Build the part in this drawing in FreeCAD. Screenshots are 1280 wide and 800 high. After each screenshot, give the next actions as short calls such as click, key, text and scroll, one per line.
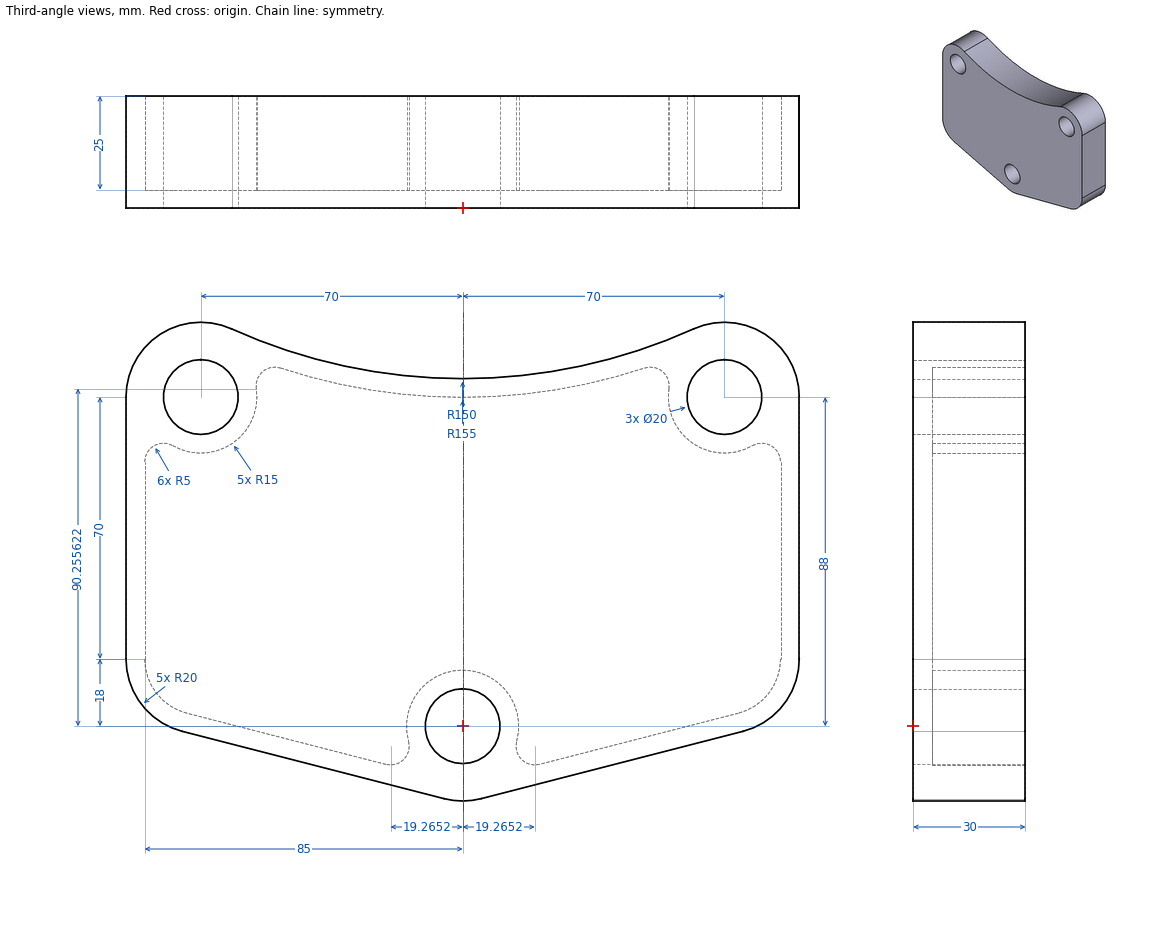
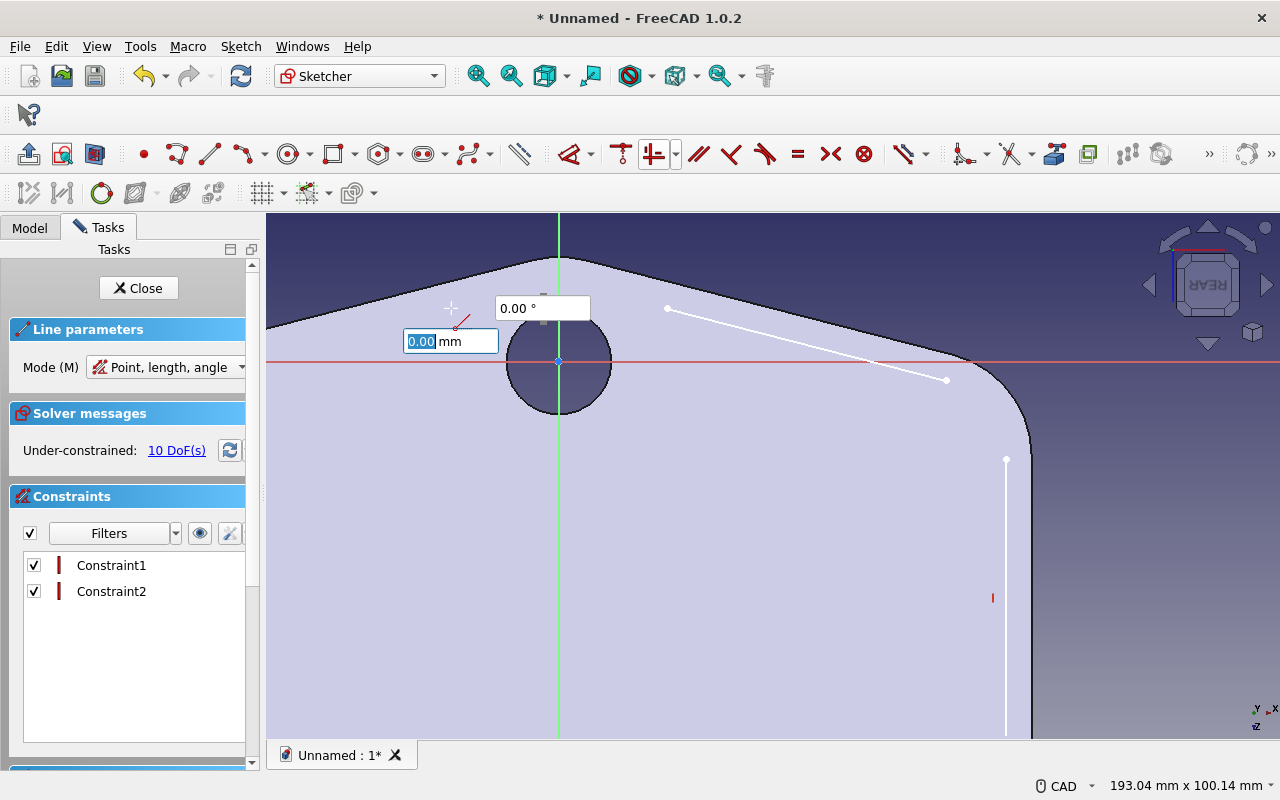
scroll(882, 341, down, 3)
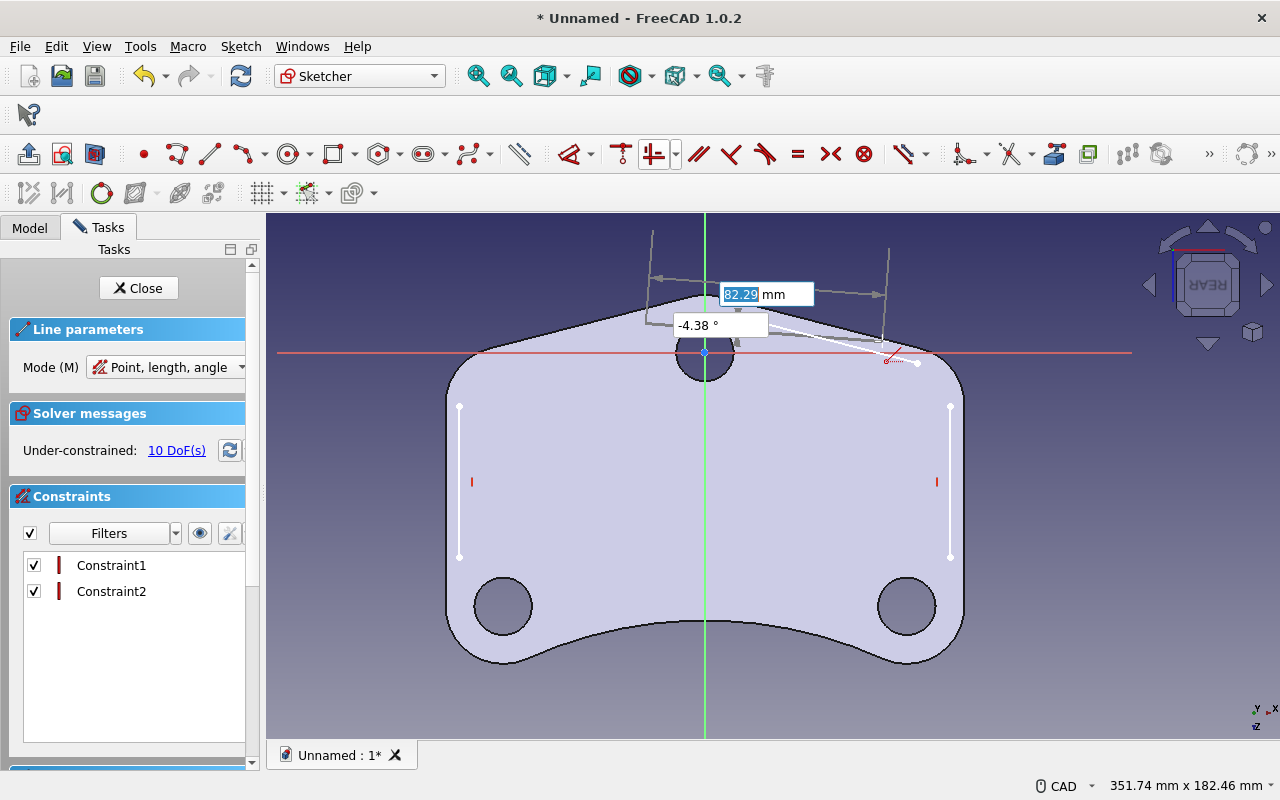
scroll(492, 363, up, 3)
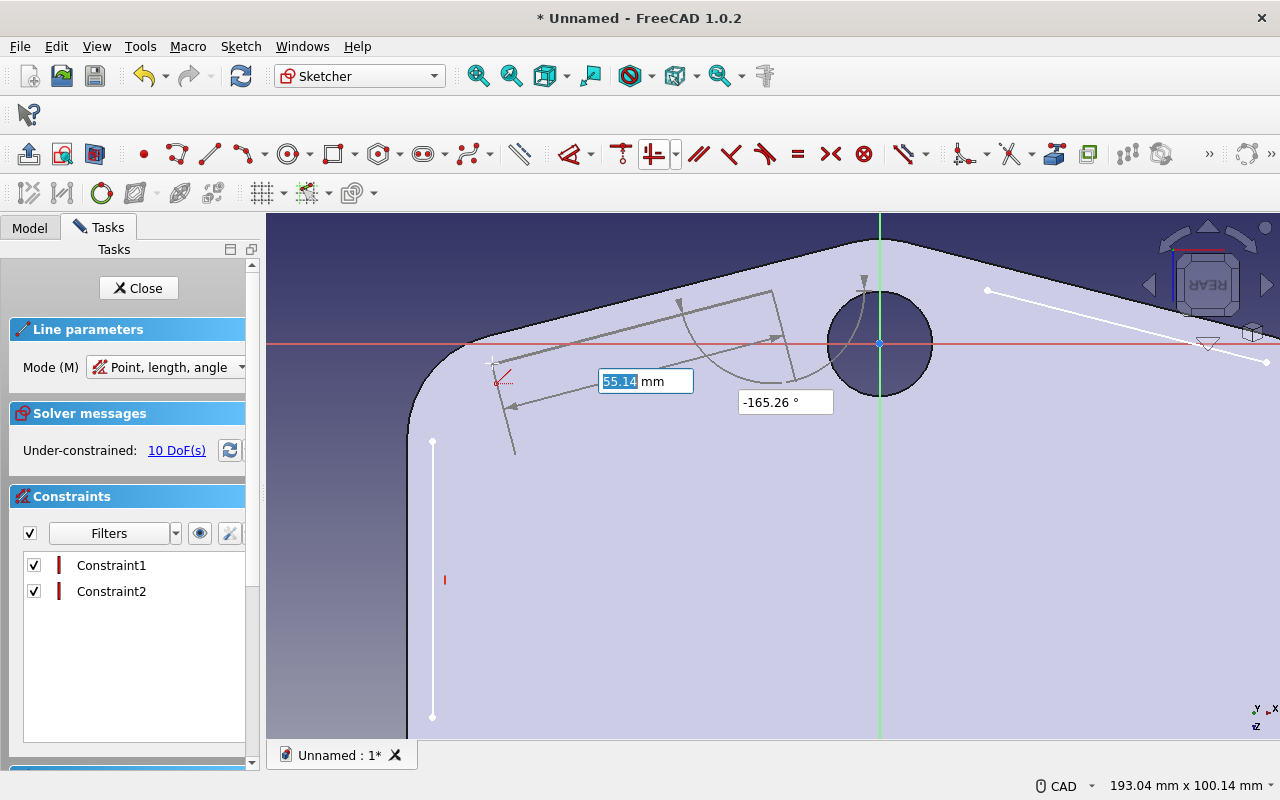
click(493, 362)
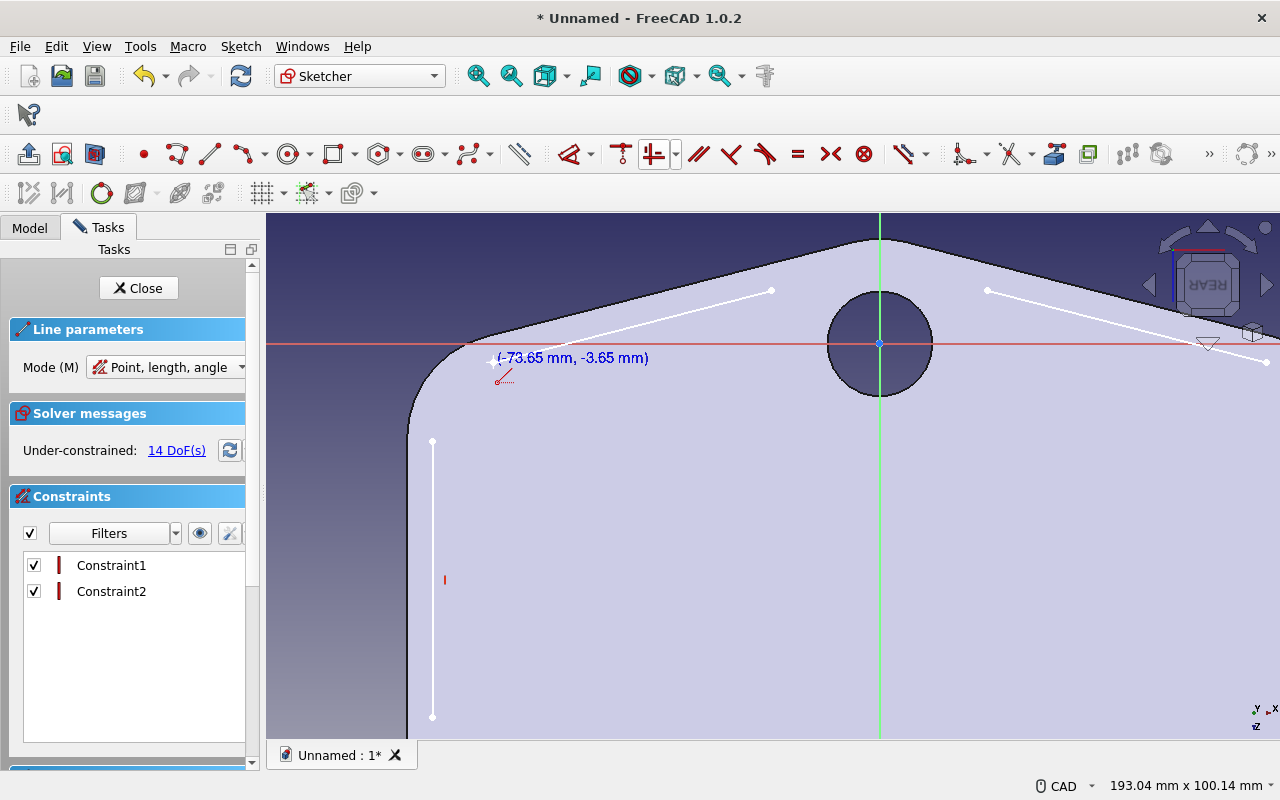
click(242, 154)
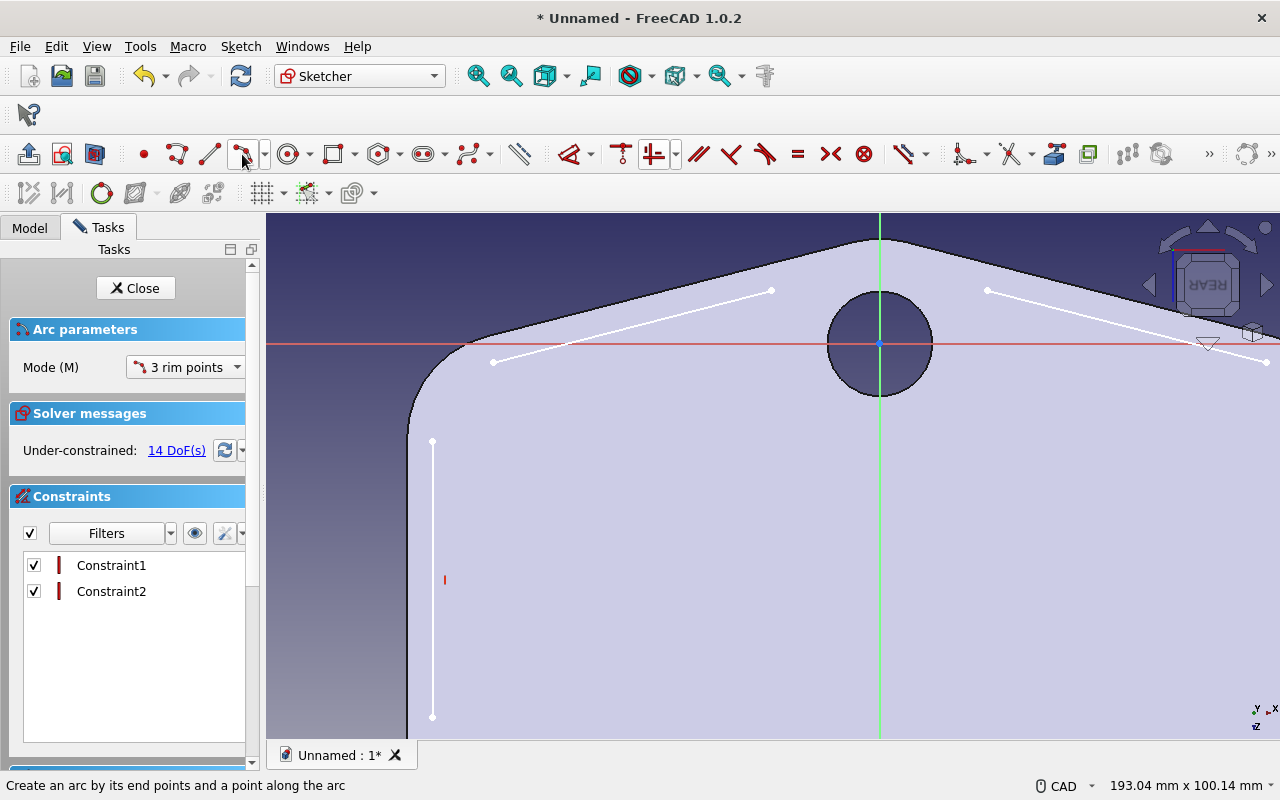
scroll(491, 363, down, 3)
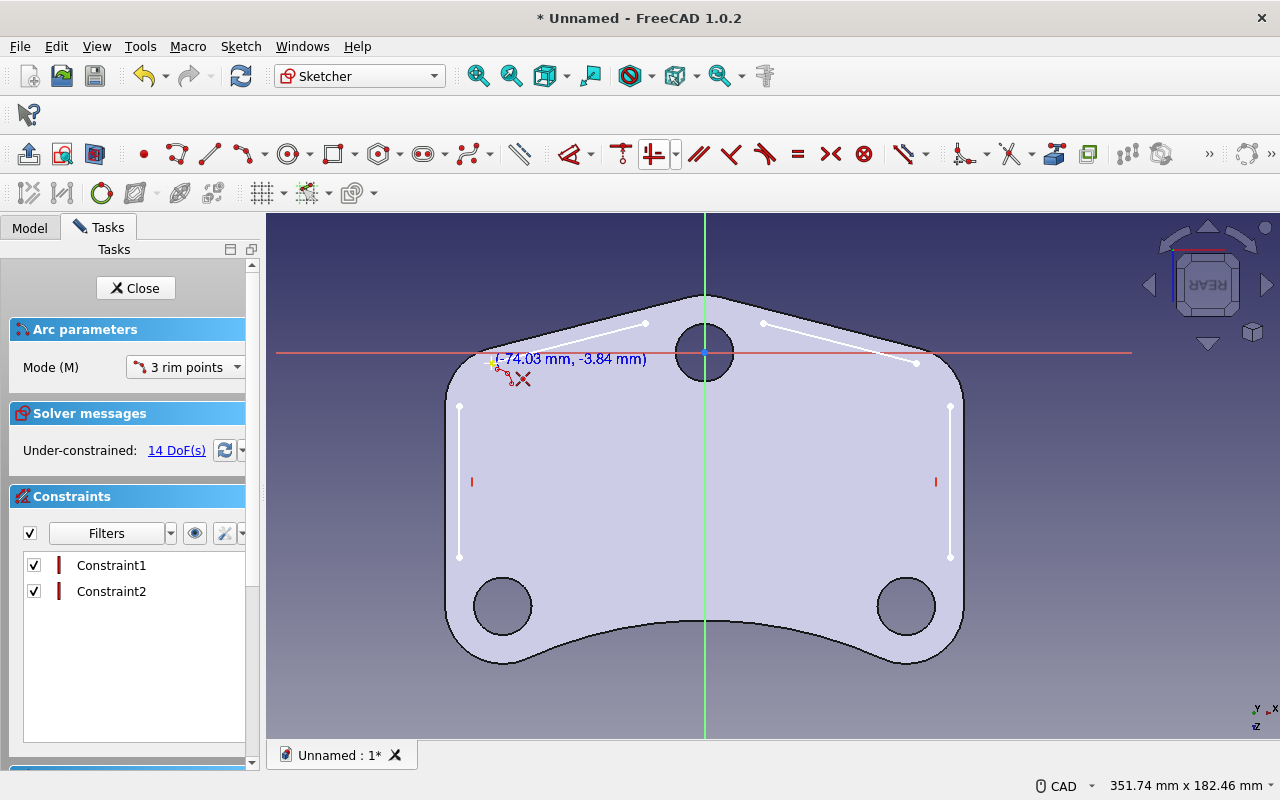
click(459, 558)
click(481, 569)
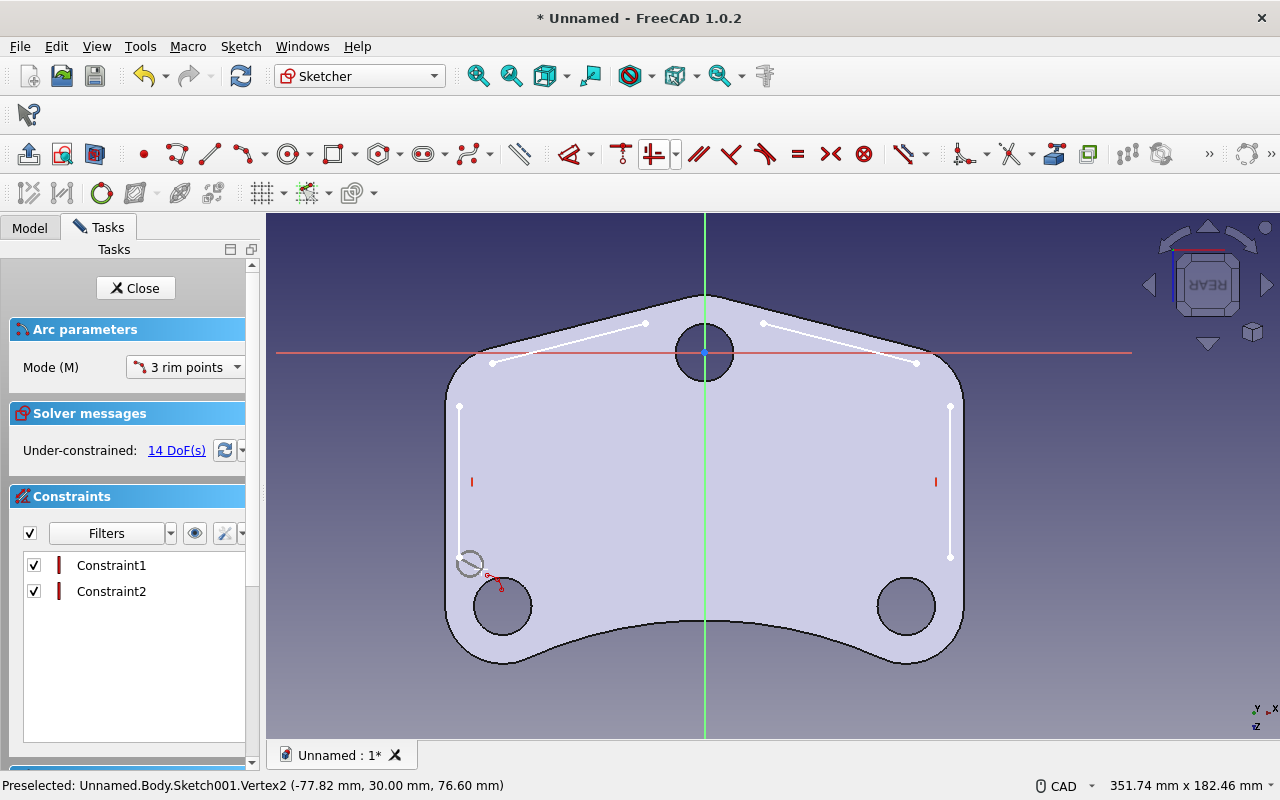
scroll(467, 569, up, 4)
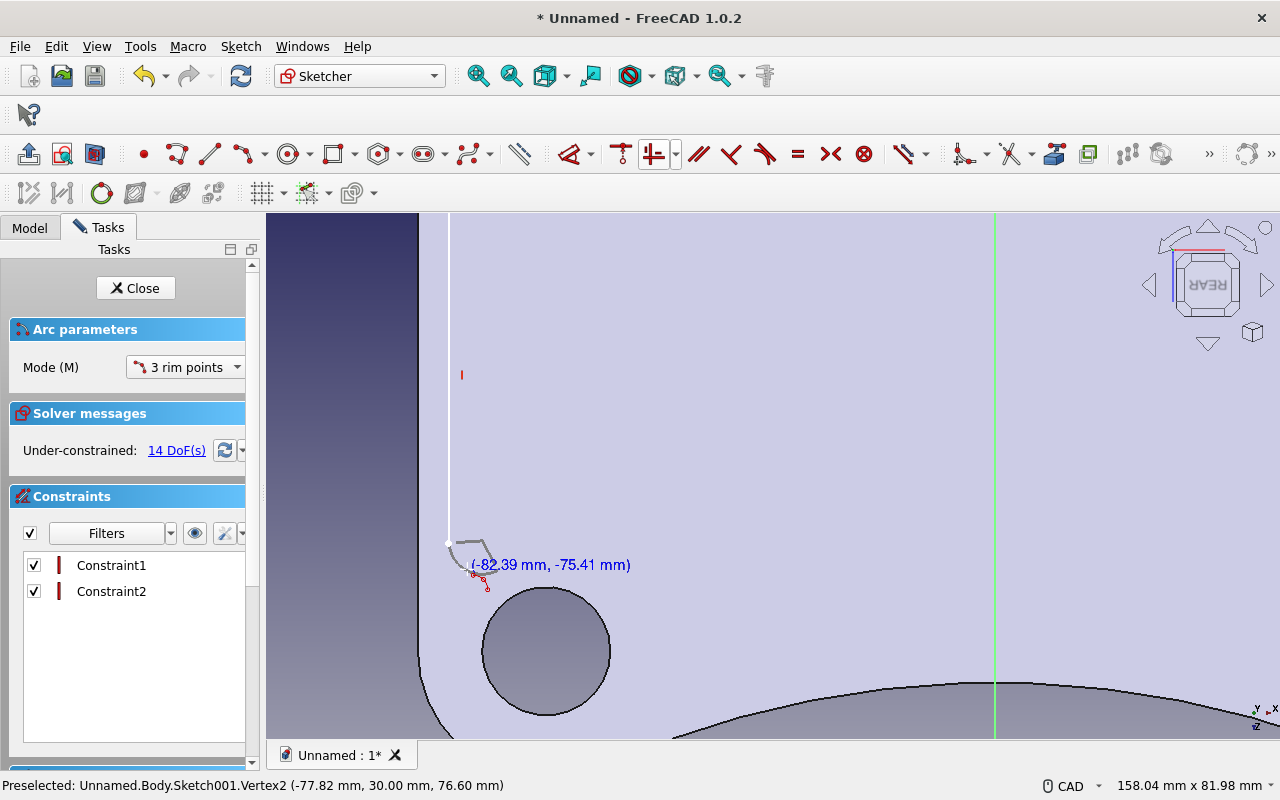
click(466, 568)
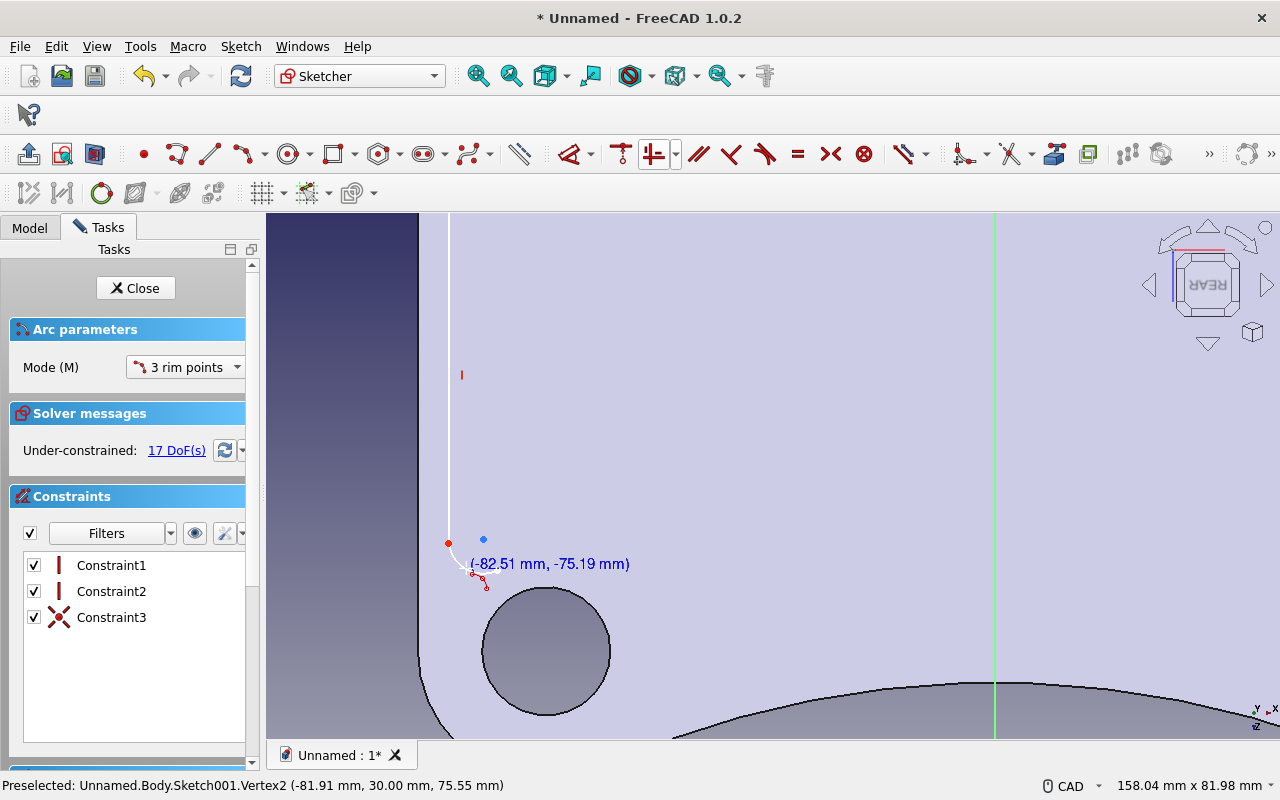
click(498, 570)
click(641, 666)
click(601, 572)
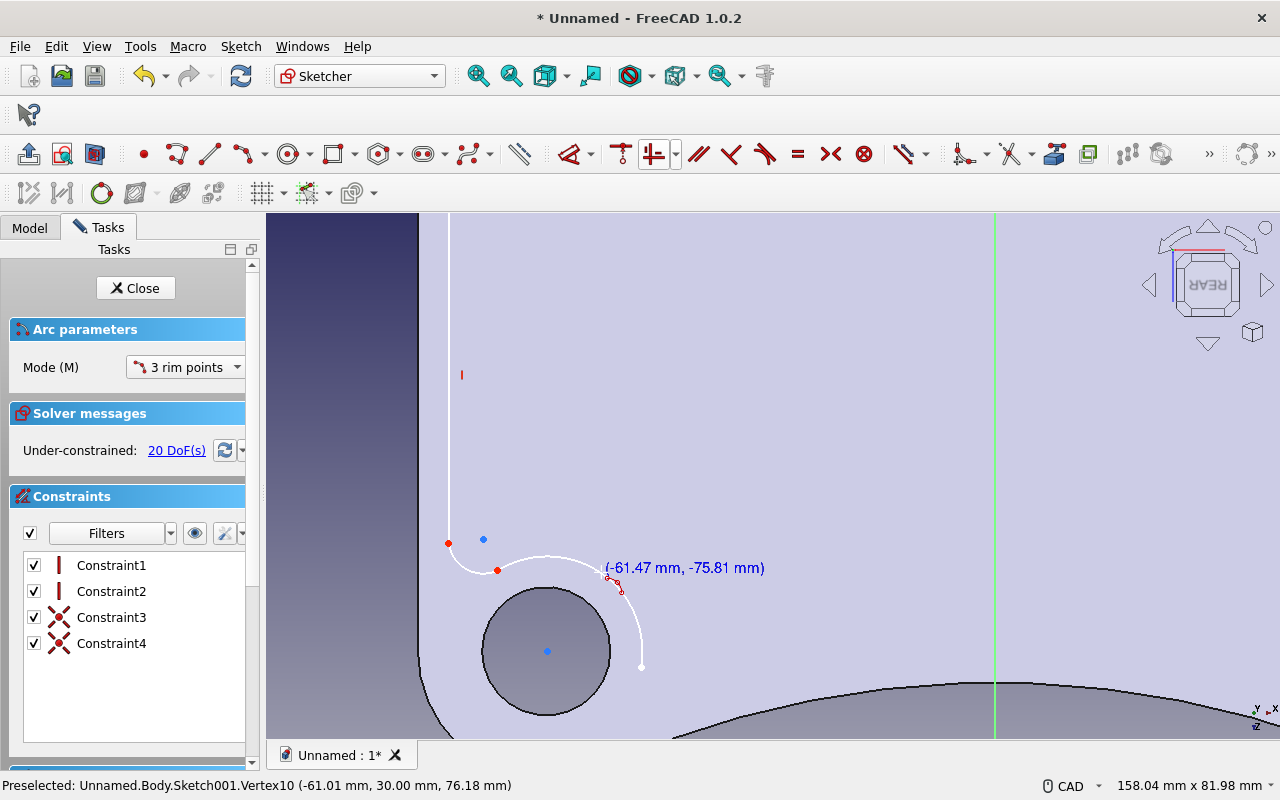
click(641, 667)
click(683, 701)
click(652, 695)